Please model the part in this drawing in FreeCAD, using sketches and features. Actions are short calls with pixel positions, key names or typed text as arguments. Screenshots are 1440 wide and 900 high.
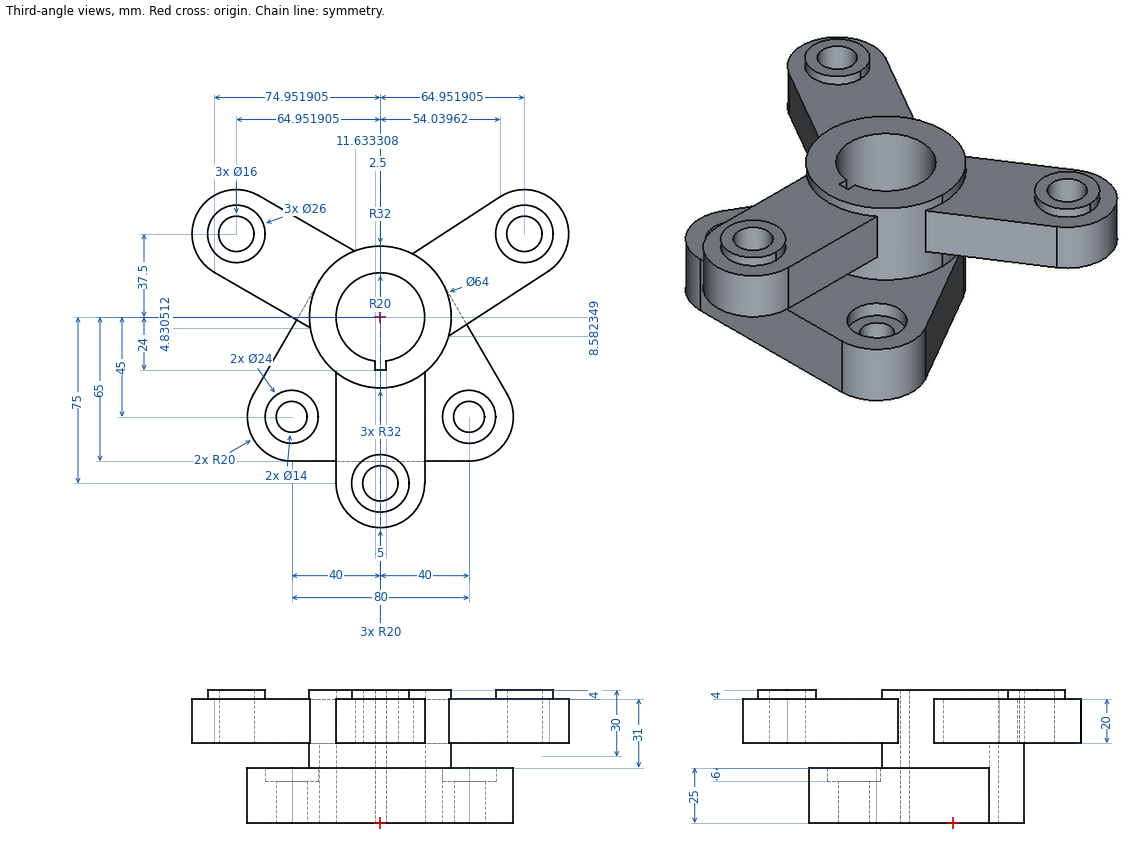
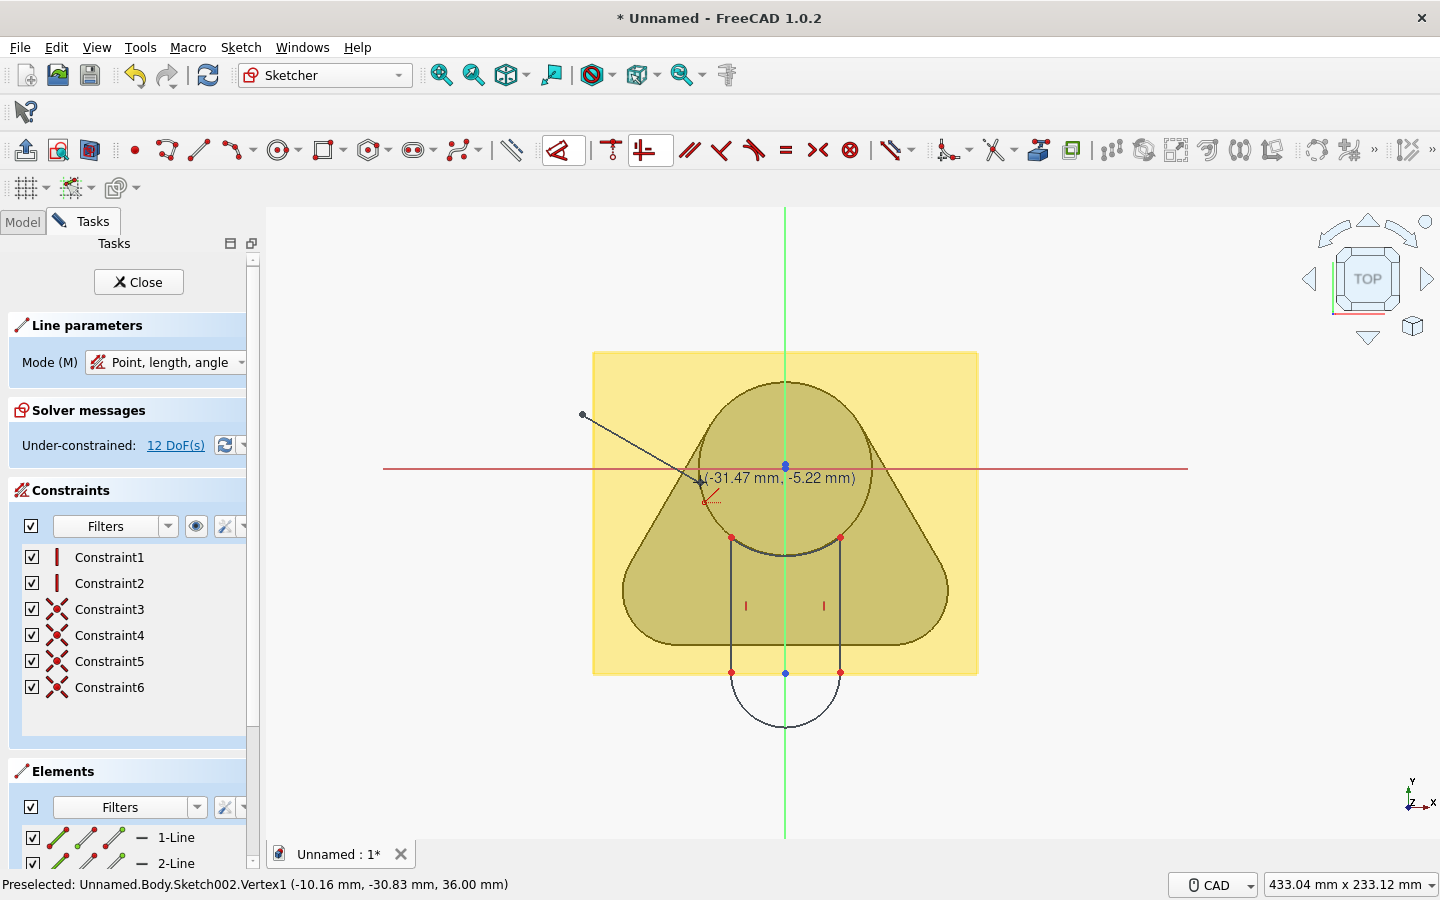
click(754, 388)
click(636, 320)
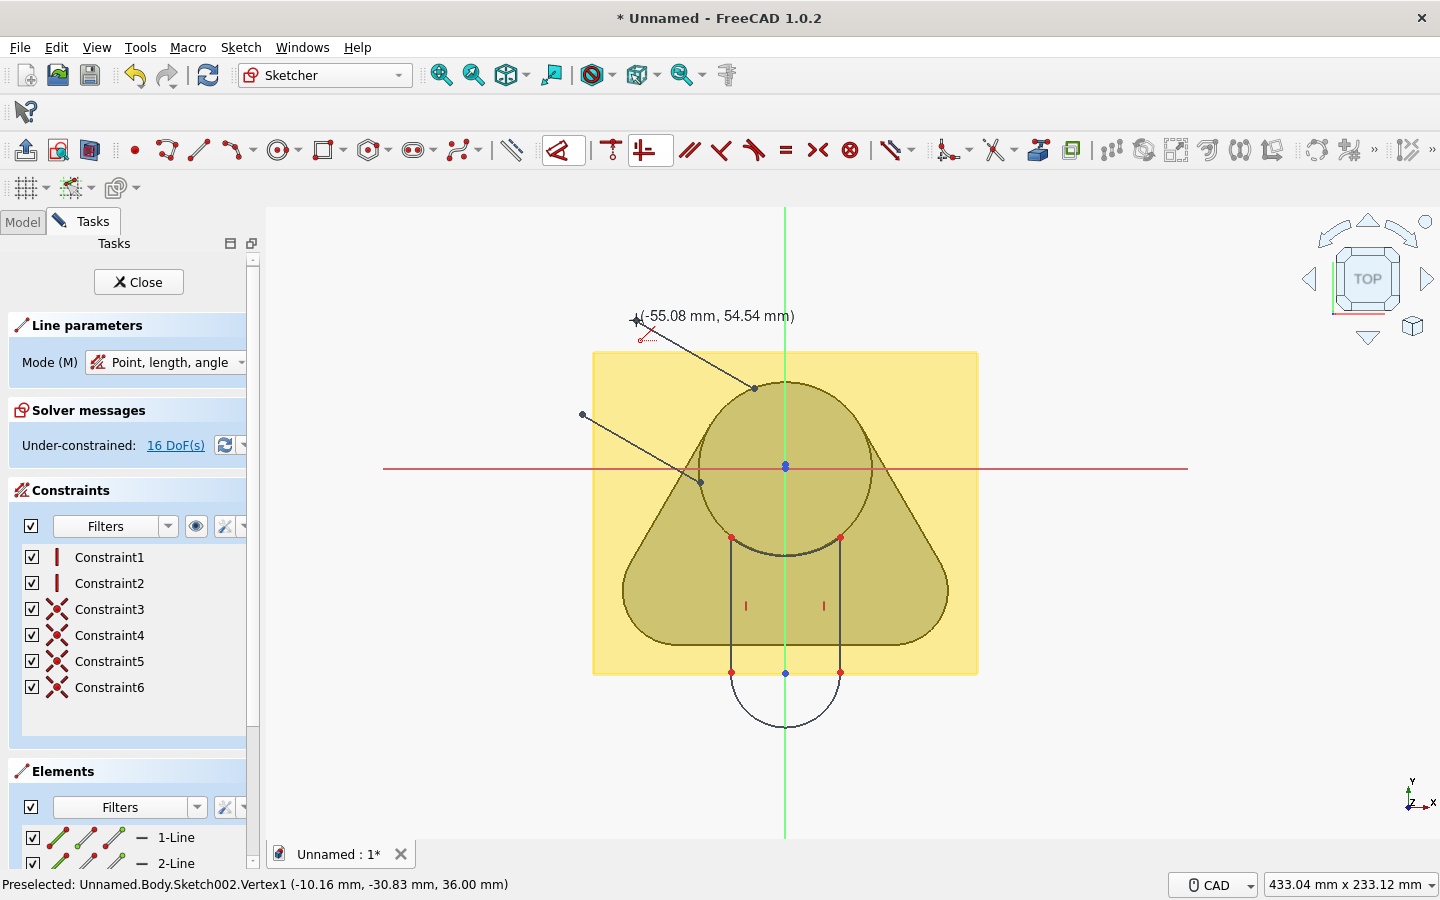
click(232, 150)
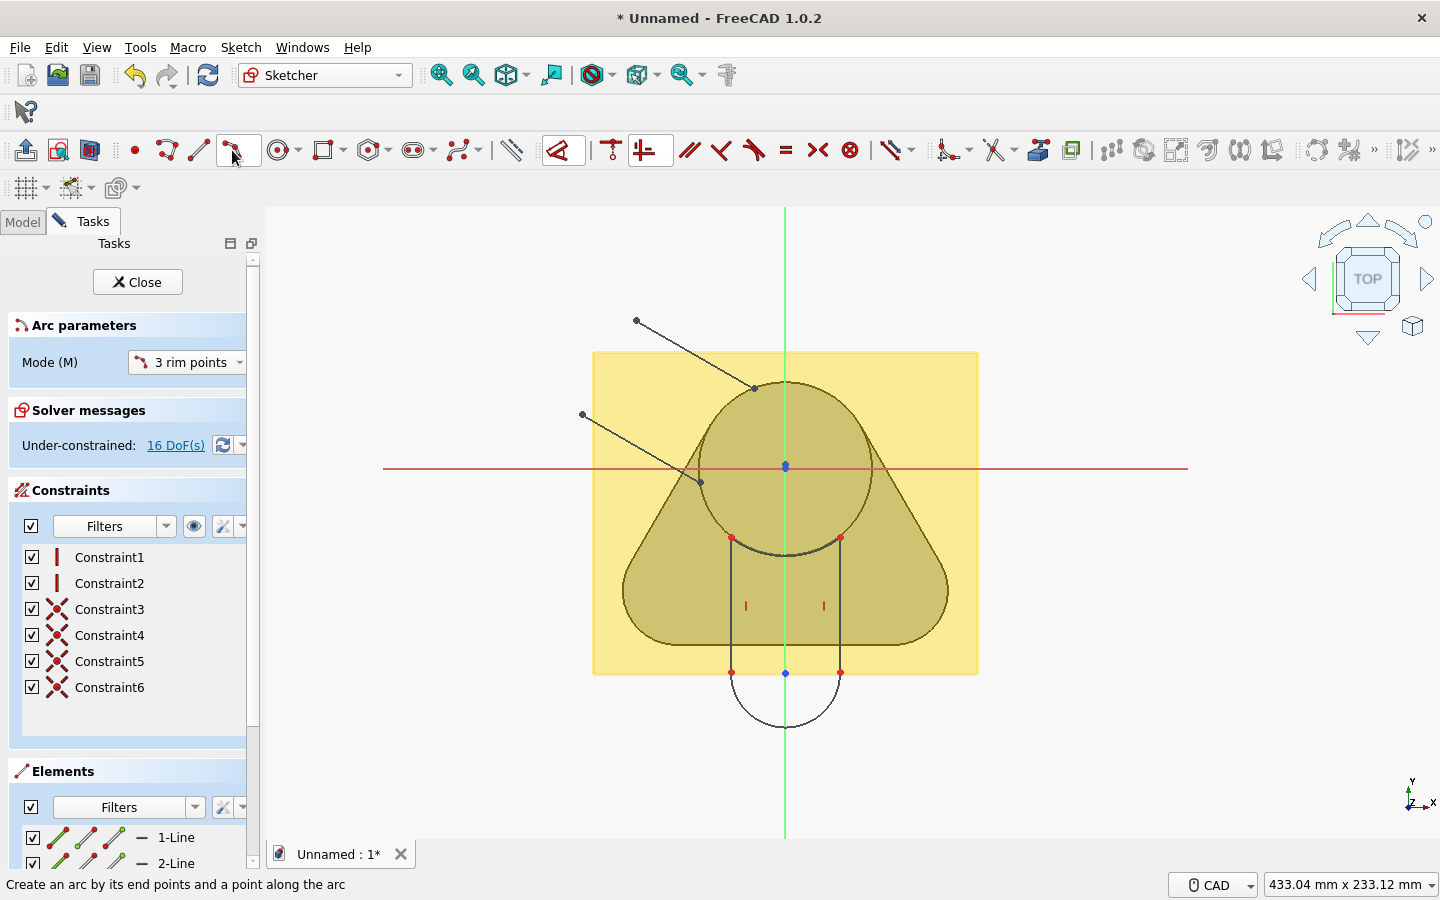
click(700, 483)
click(754, 389)
click(710, 425)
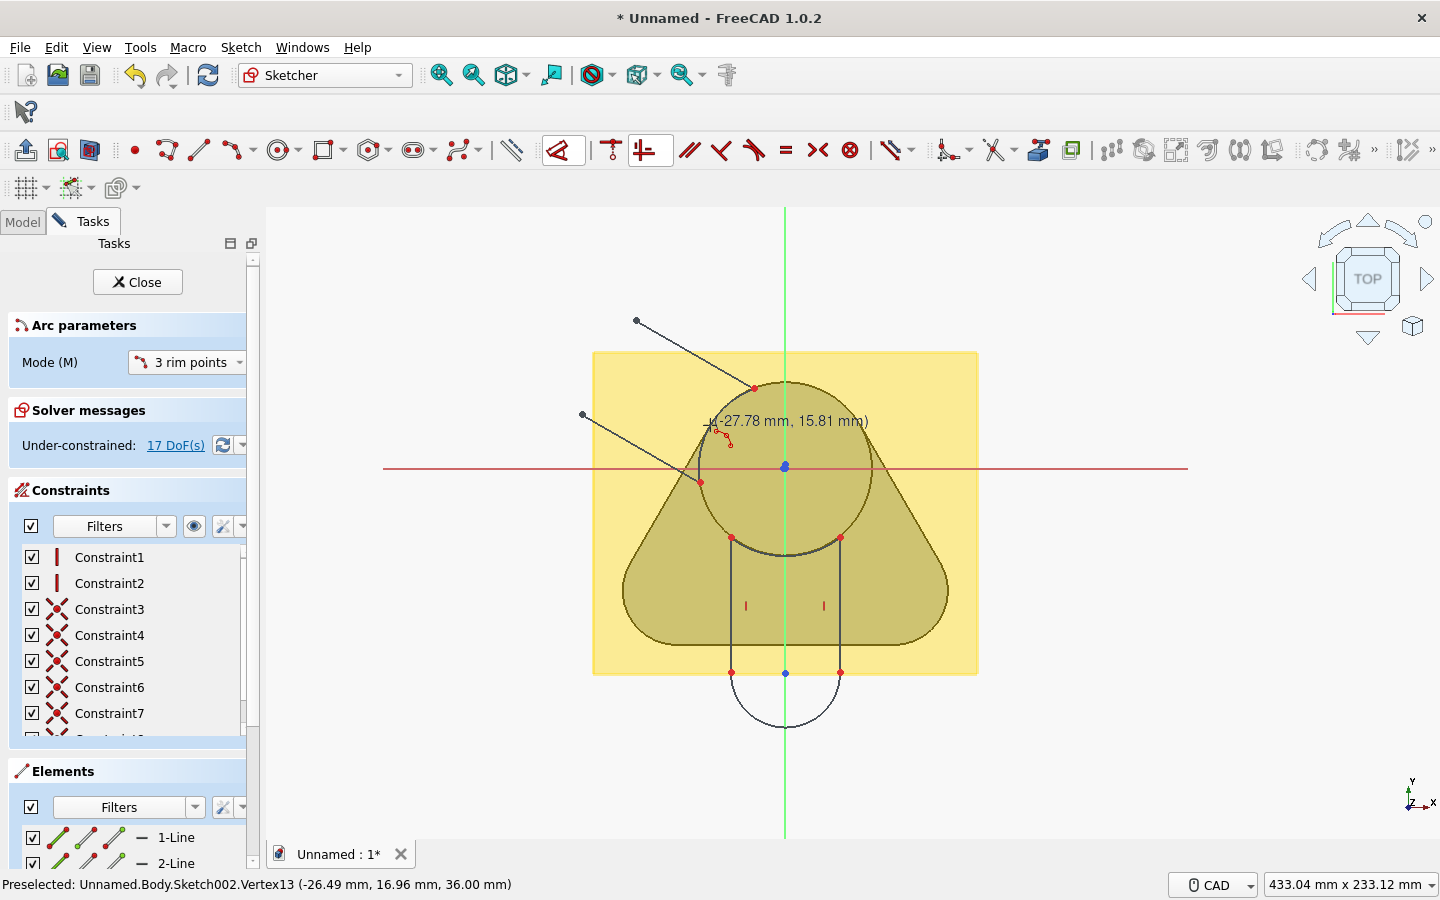
click(636, 321)
click(582, 415)
click(562, 340)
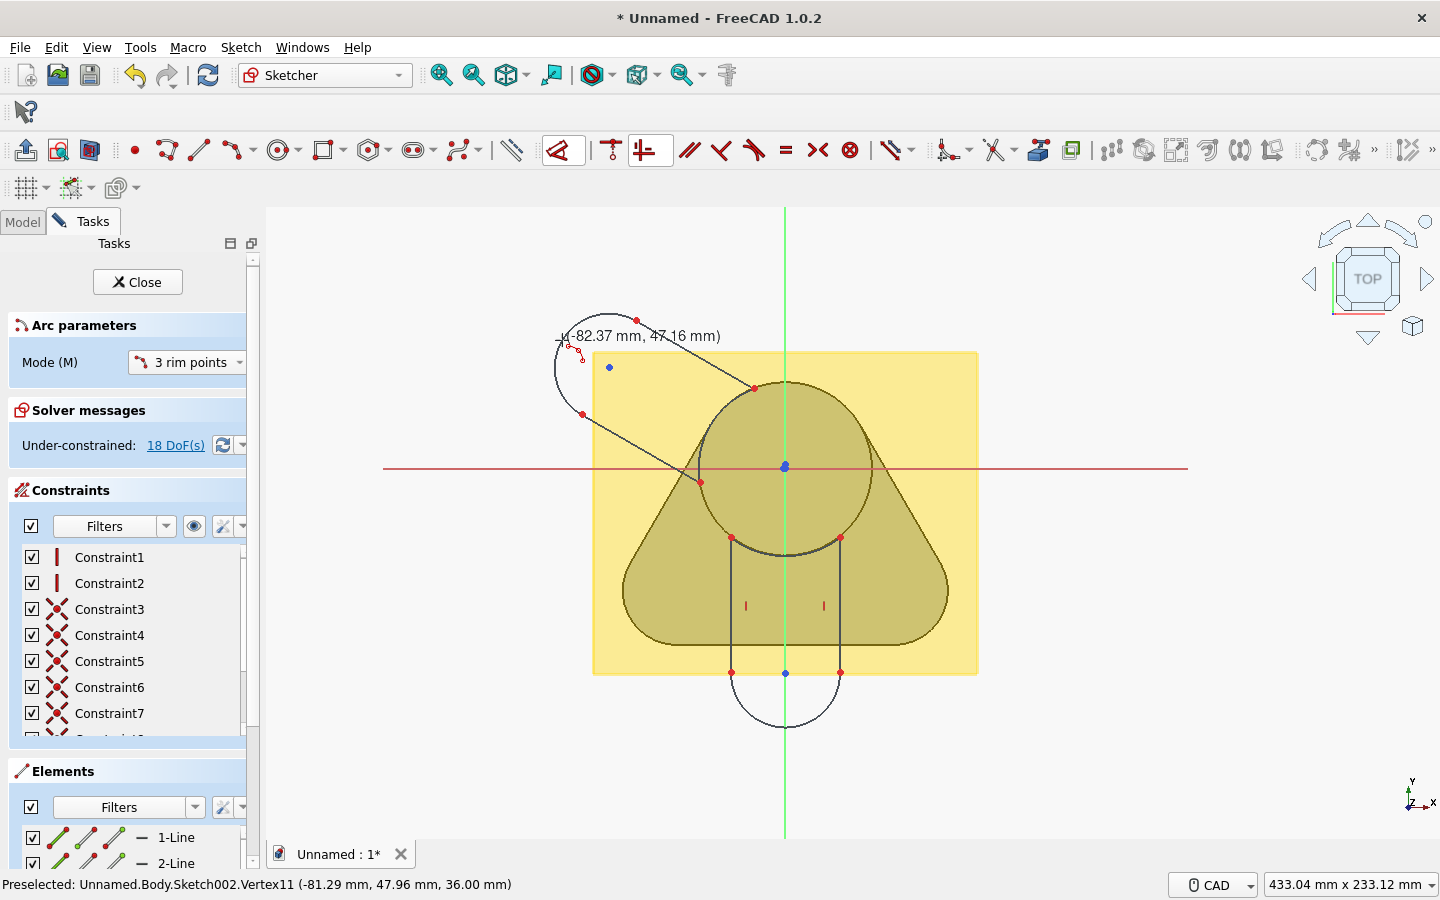
click(200, 150)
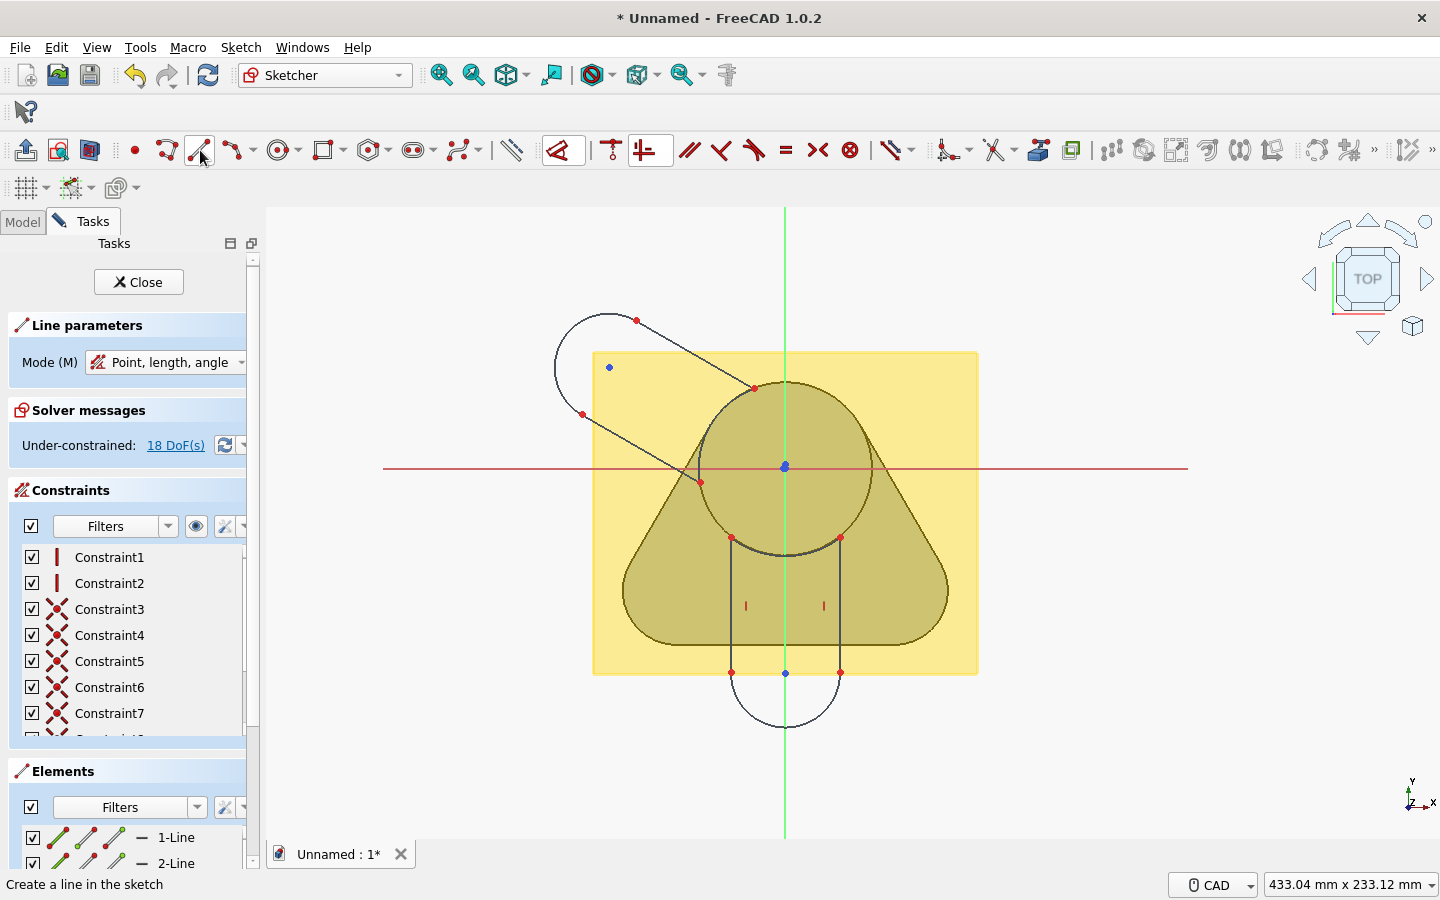
click(932, 322)
click(825, 392)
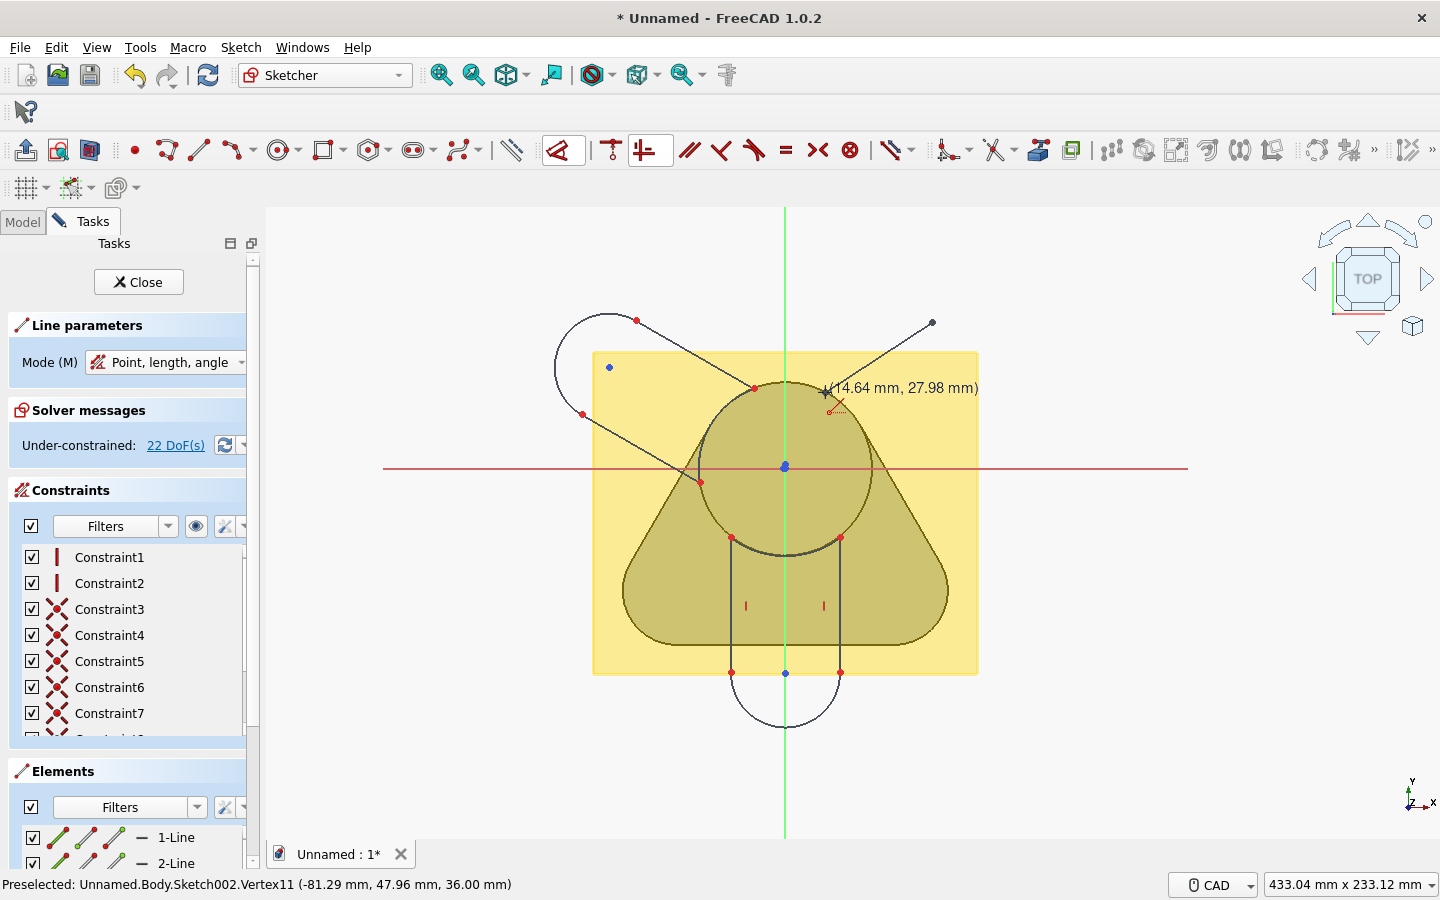
click(869, 492)
click(991, 413)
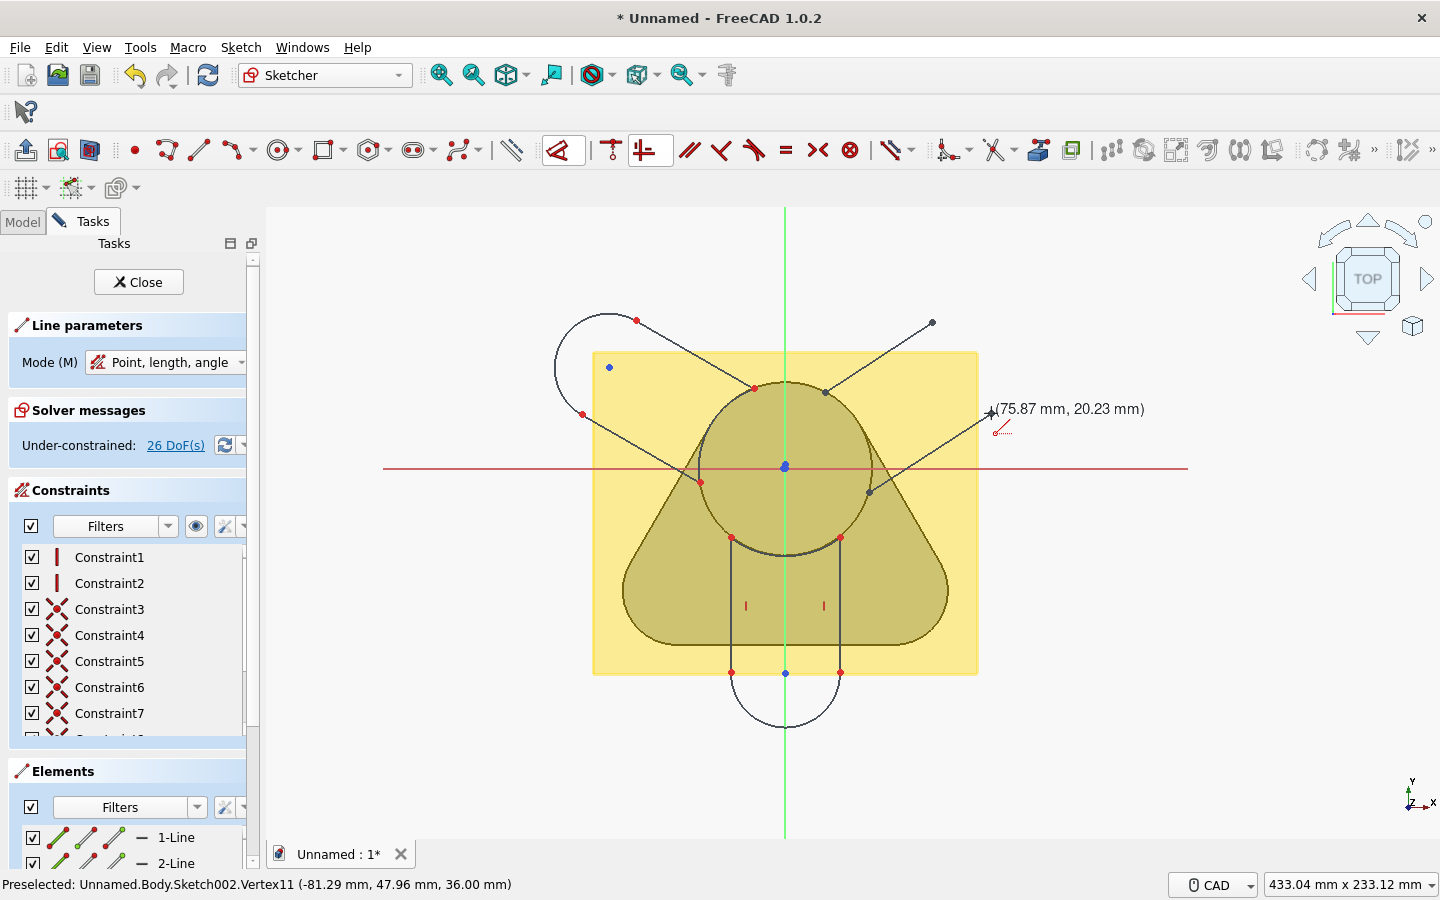
click(232, 150)